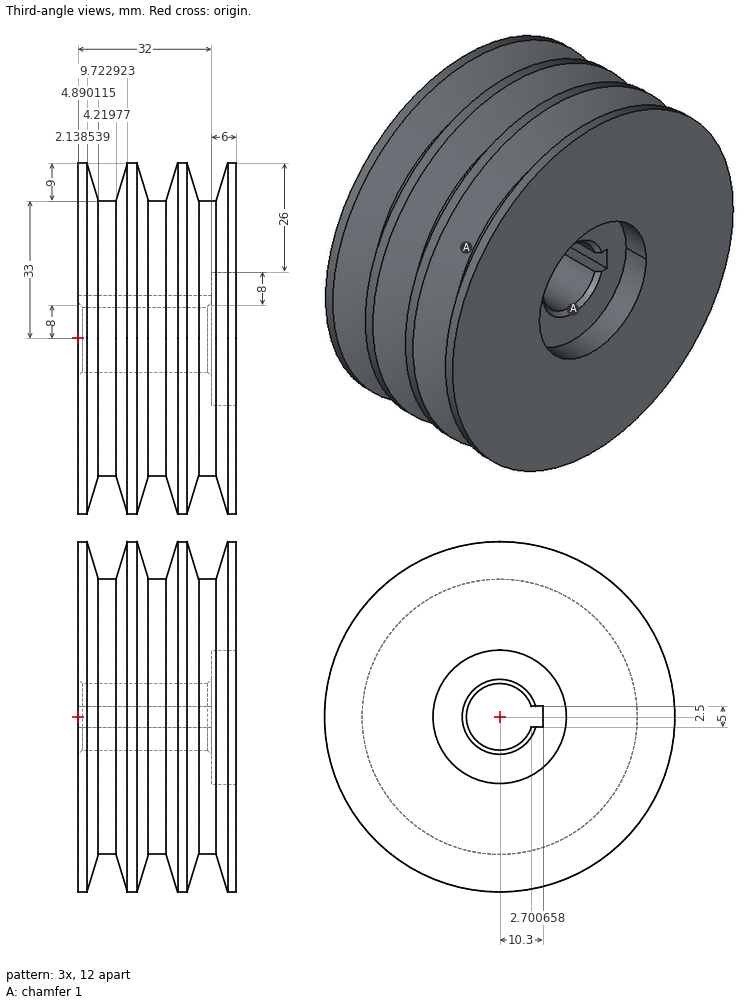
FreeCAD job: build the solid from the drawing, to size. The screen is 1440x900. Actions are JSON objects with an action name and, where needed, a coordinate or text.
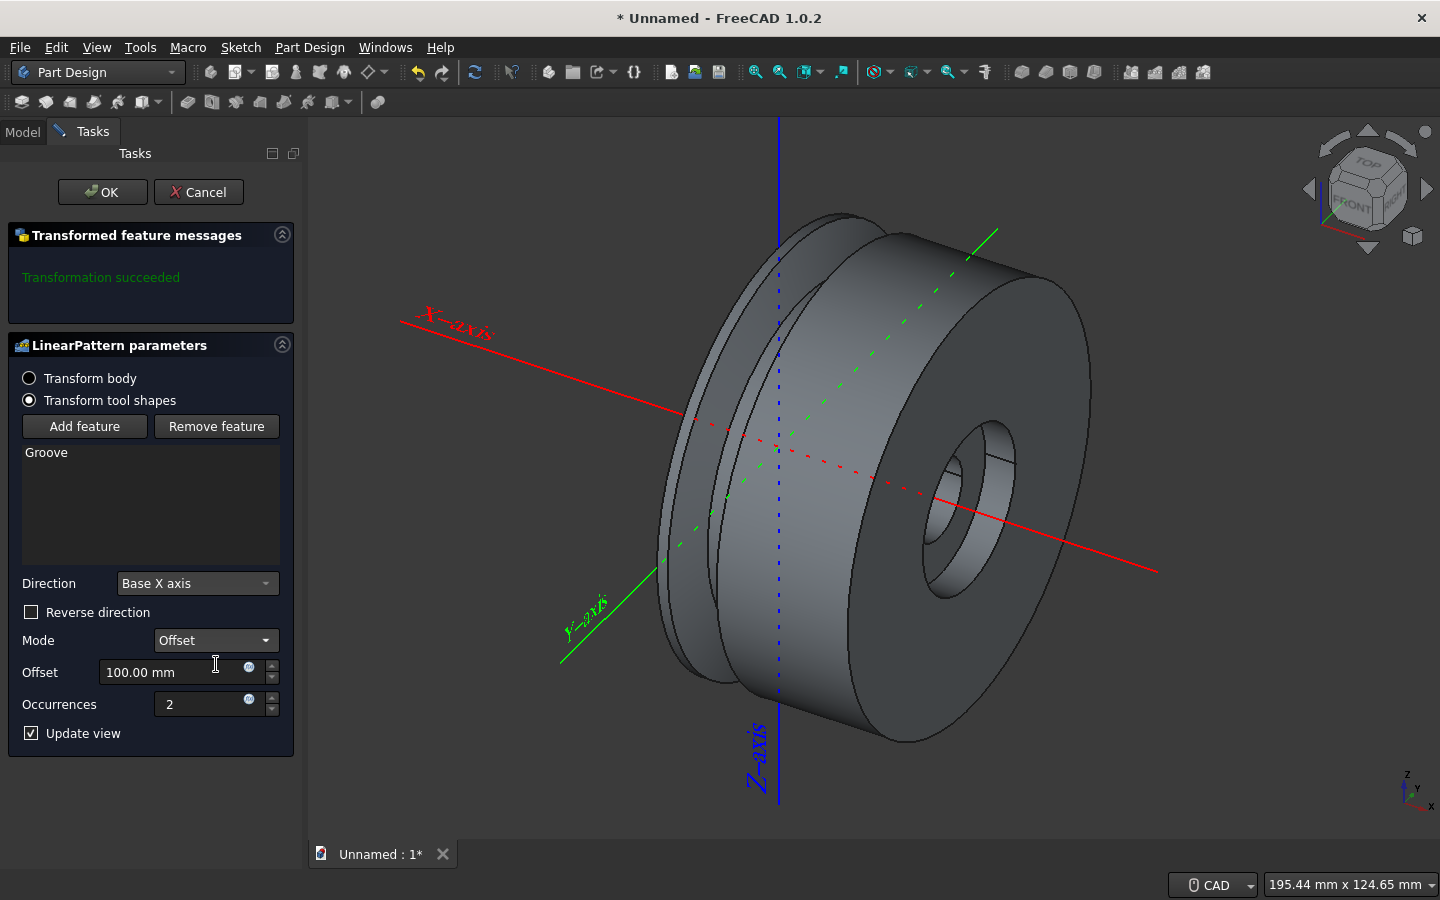
{"action": "triple_click", "coordinate": [182, 672]}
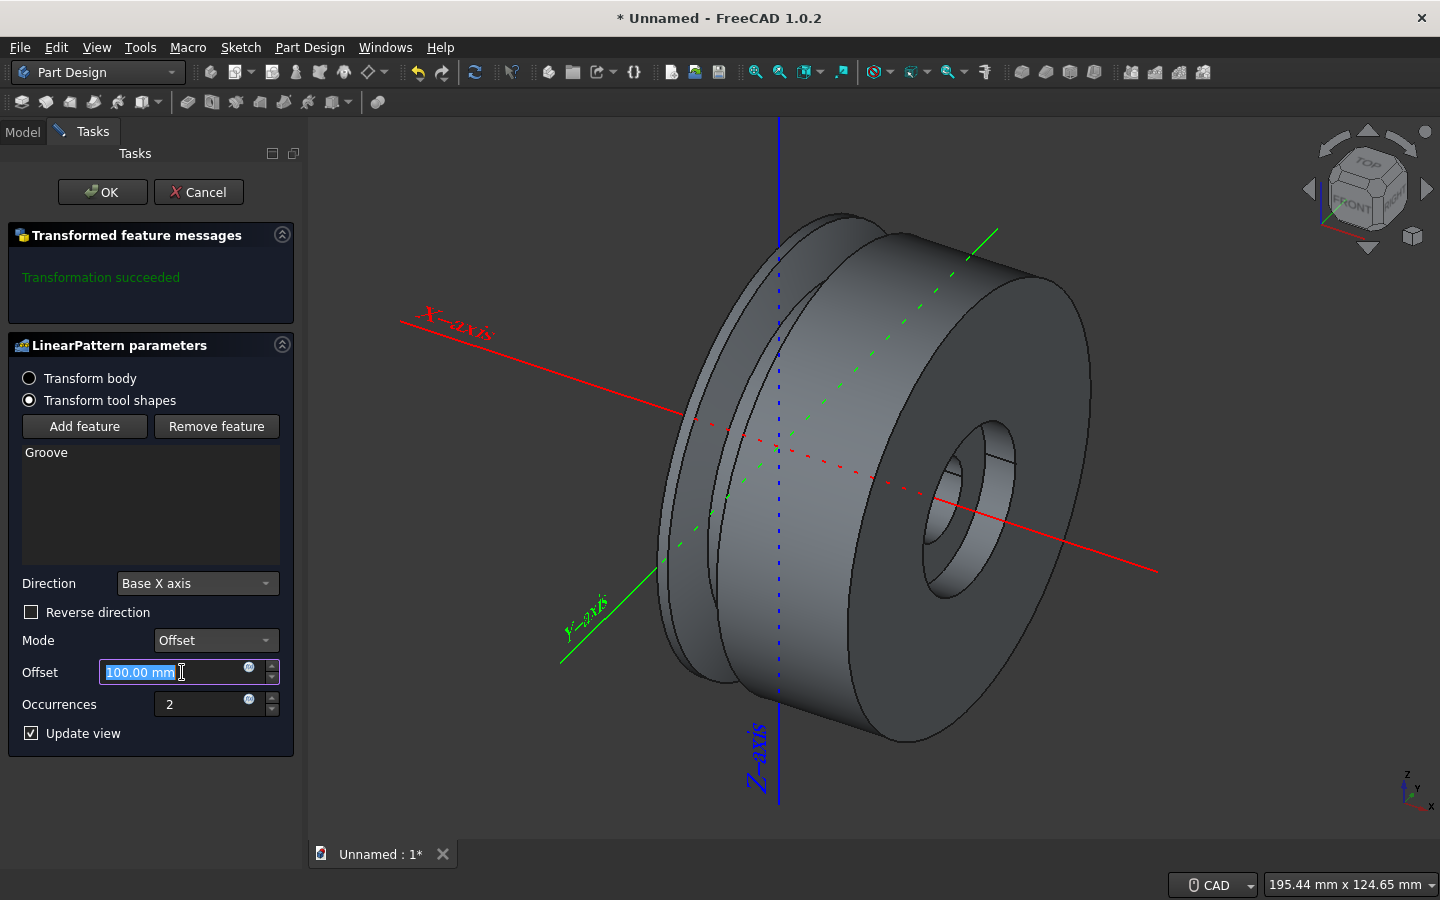
{"action": "type", "text": "12"}
{"action": "key", "text": "Tab"}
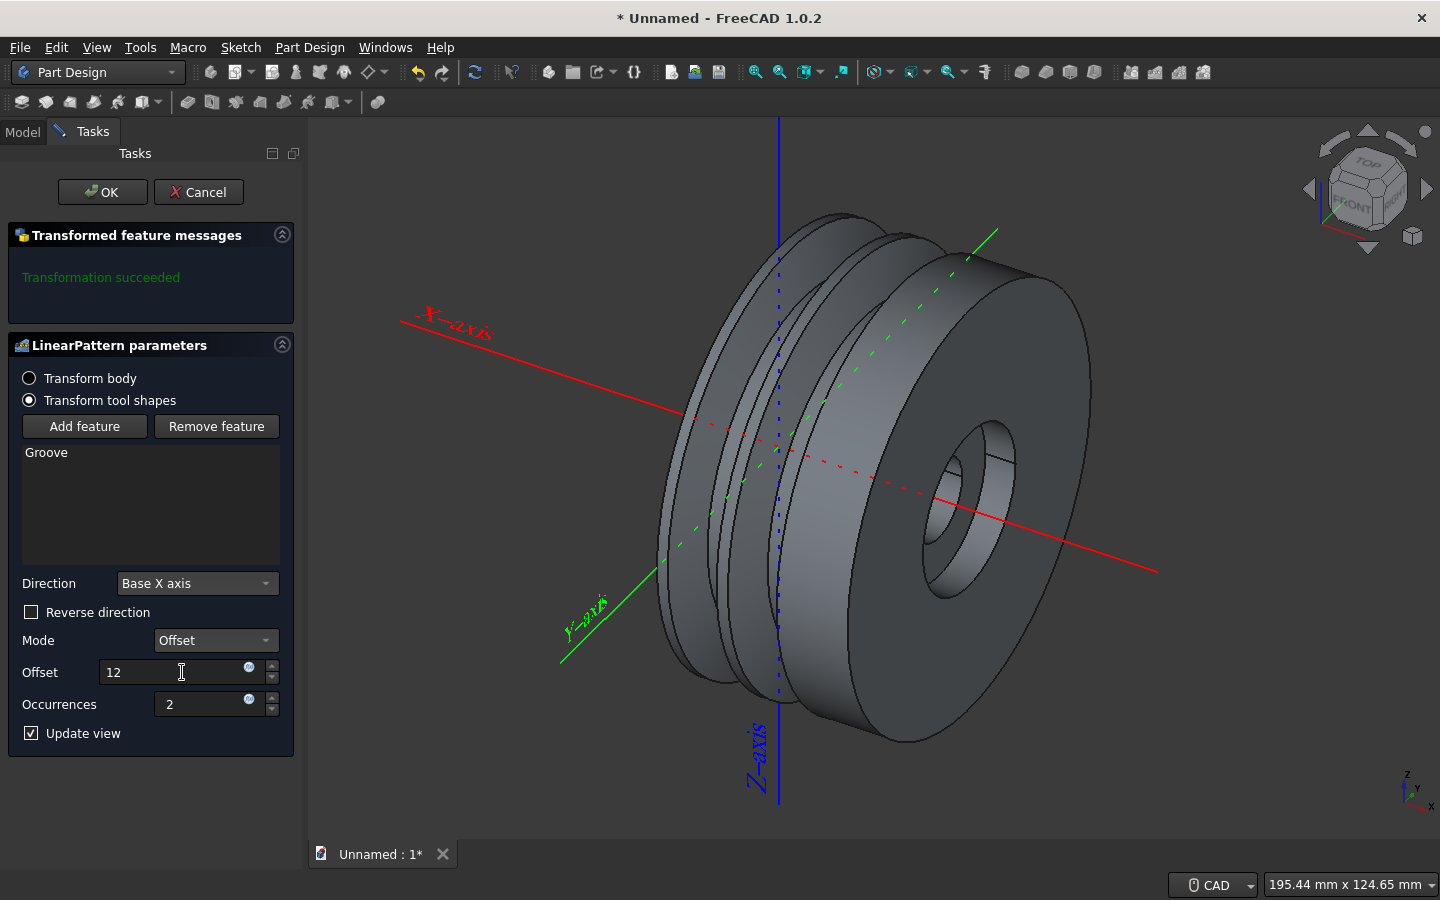
{"action": "triple_click", "coordinate": [209, 704]}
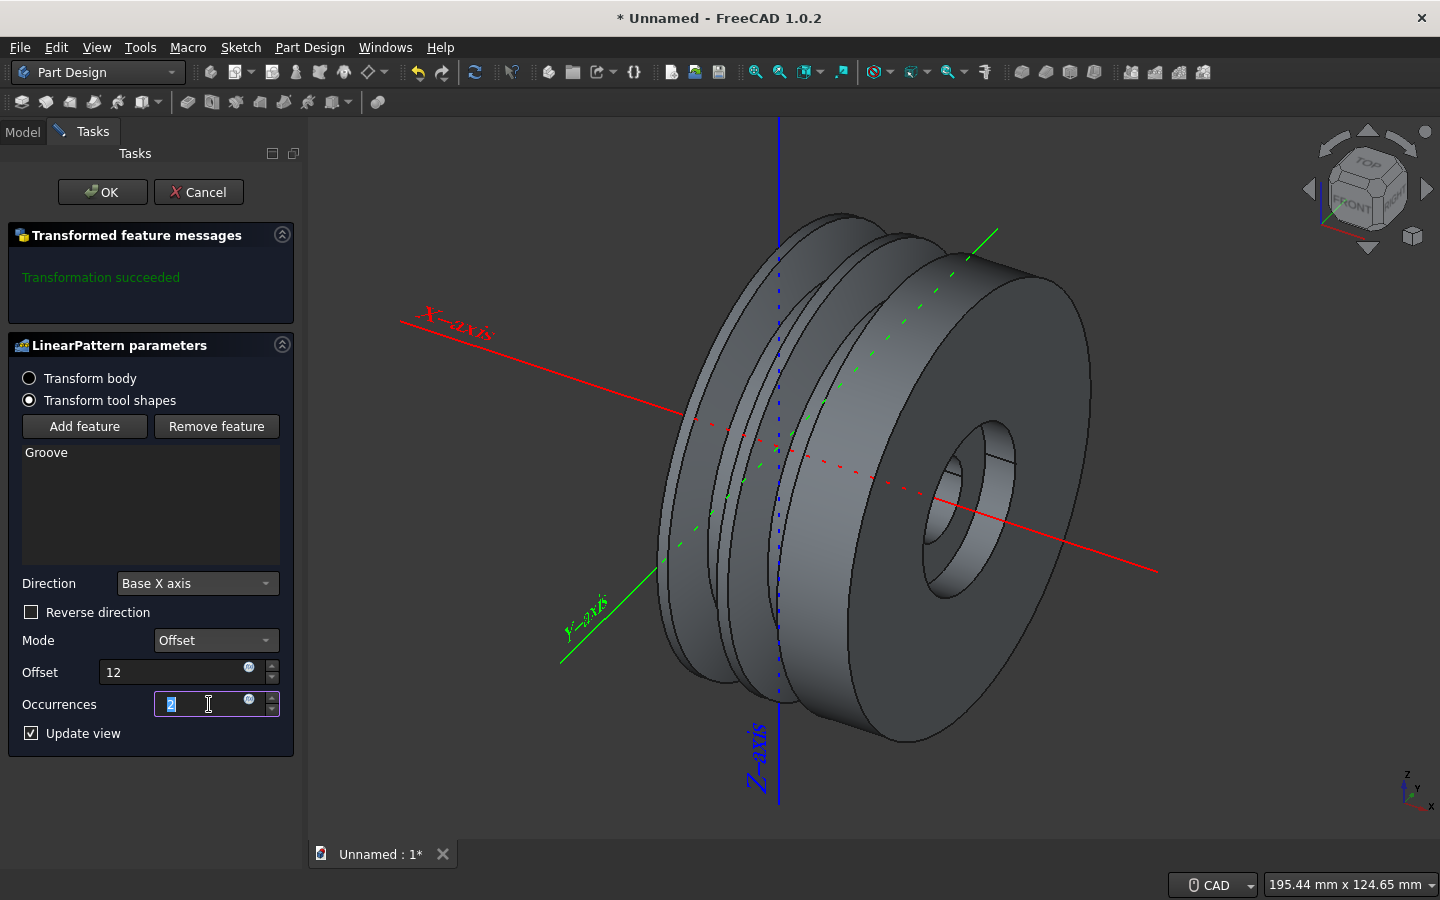
{"action": "type", "text": "3"}
{"action": "key", "text": "Tab"}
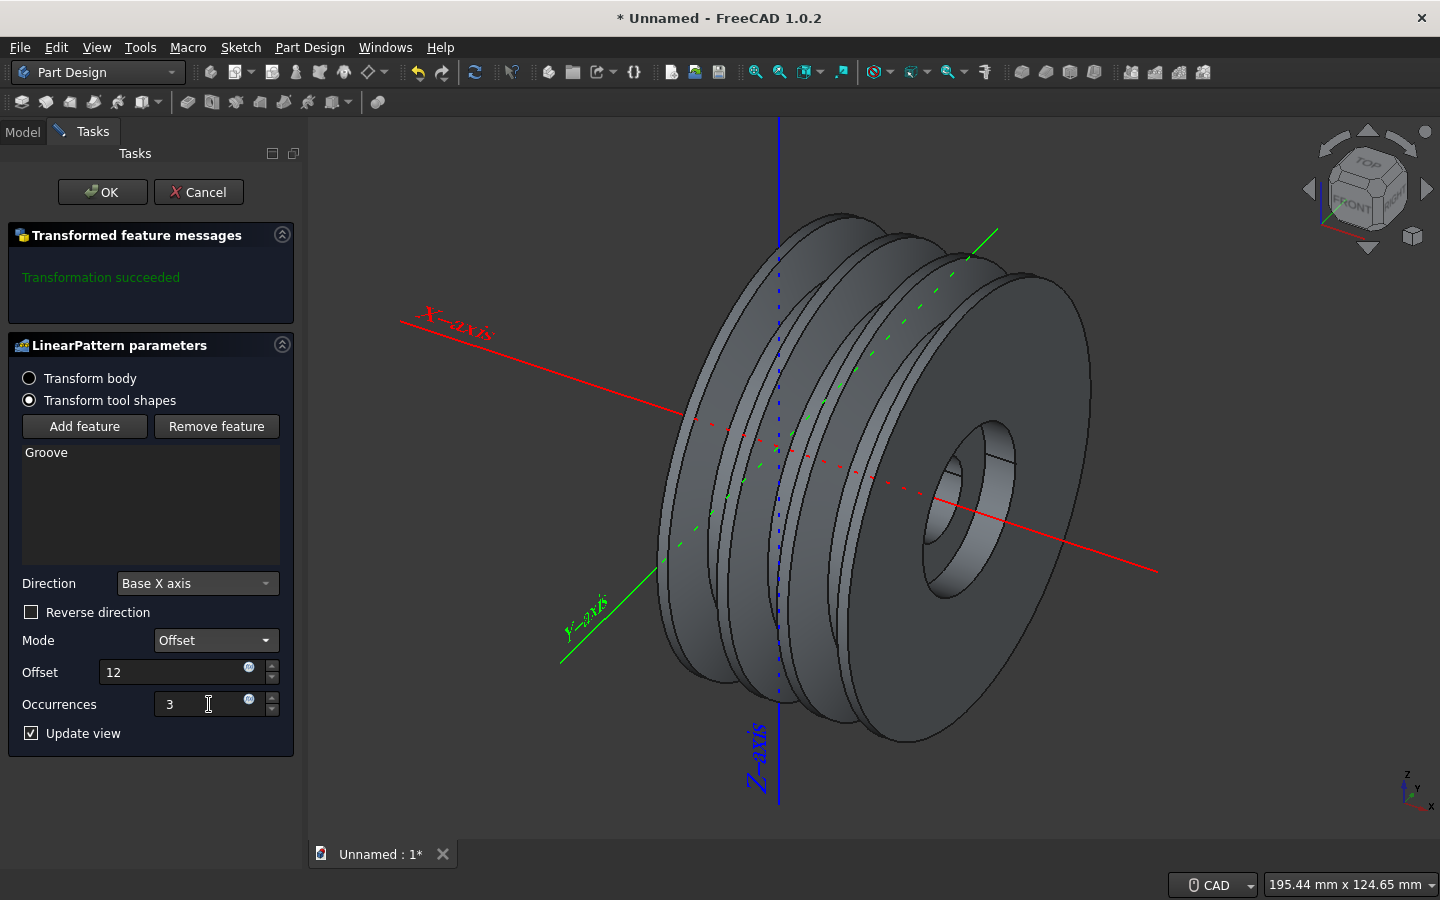
{"action": "left_click", "coordinate": [103, 192]}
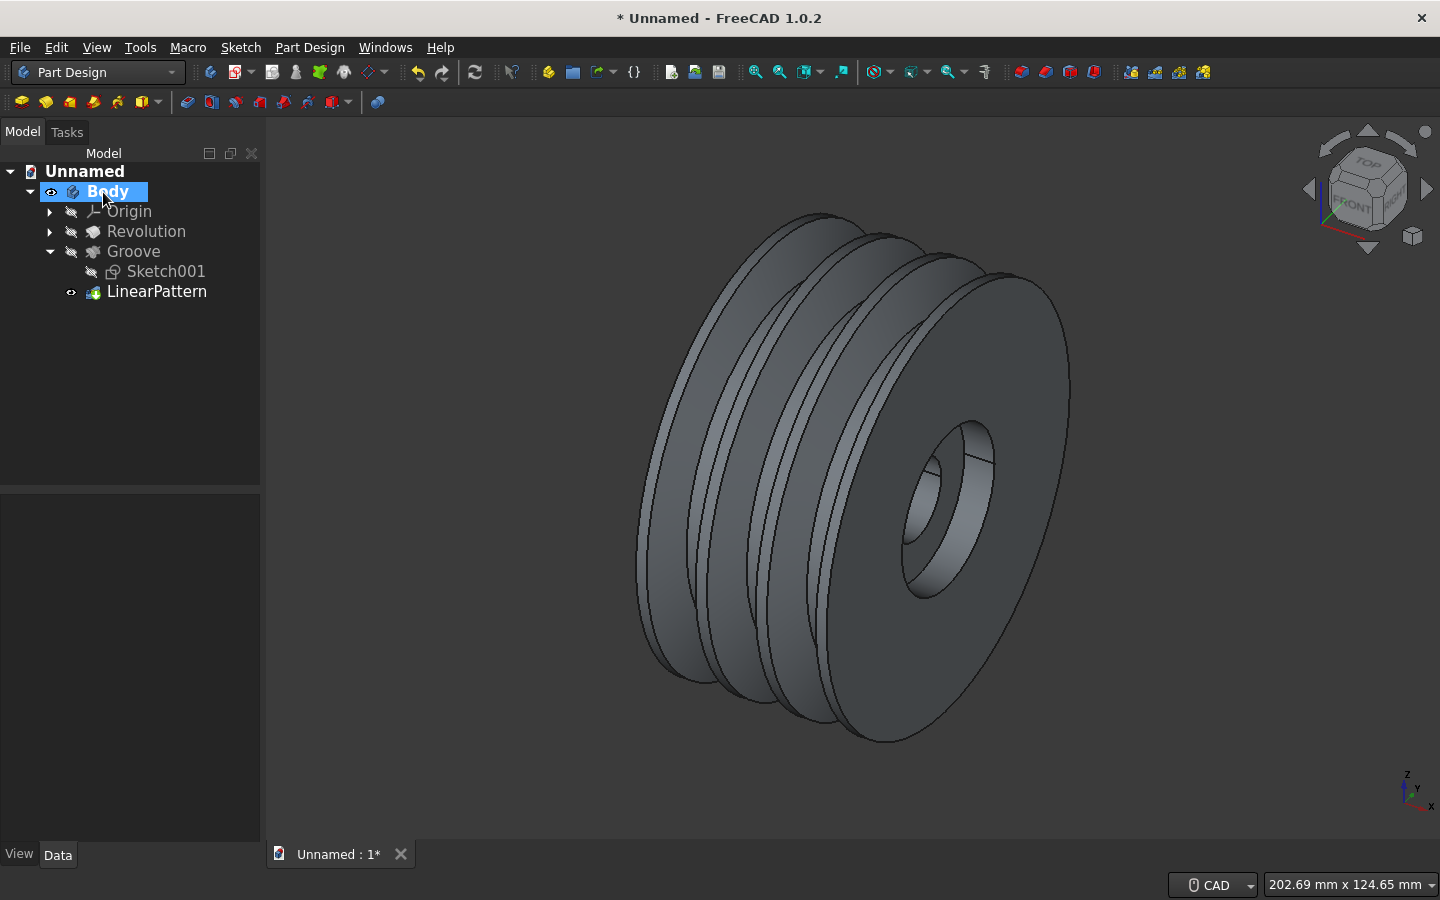
{"action": "left_click", "coordinate": [911, 542]}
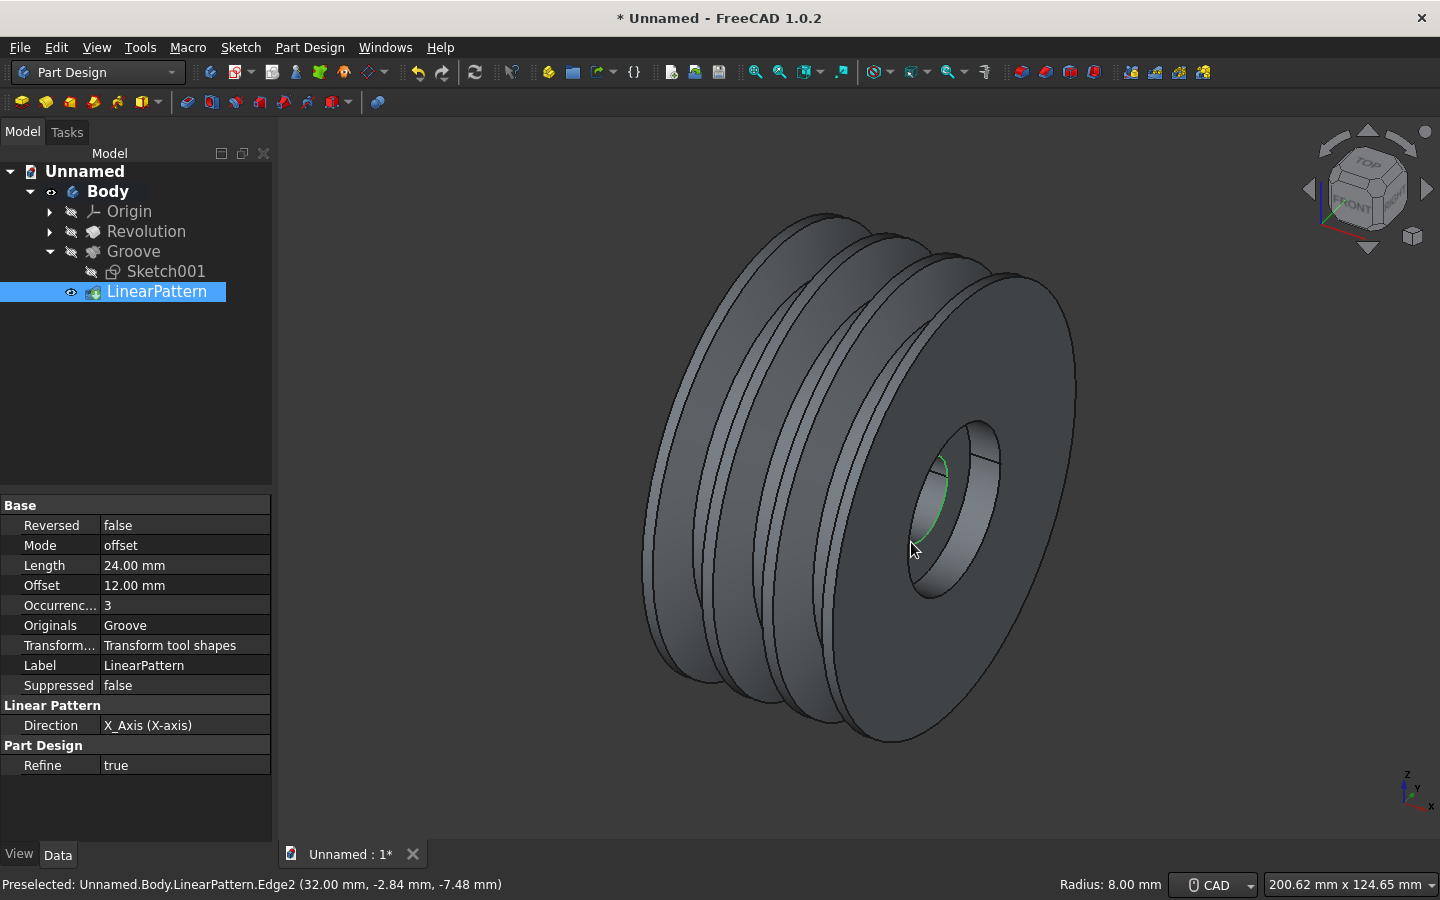
{"action": "key", "text": "0"}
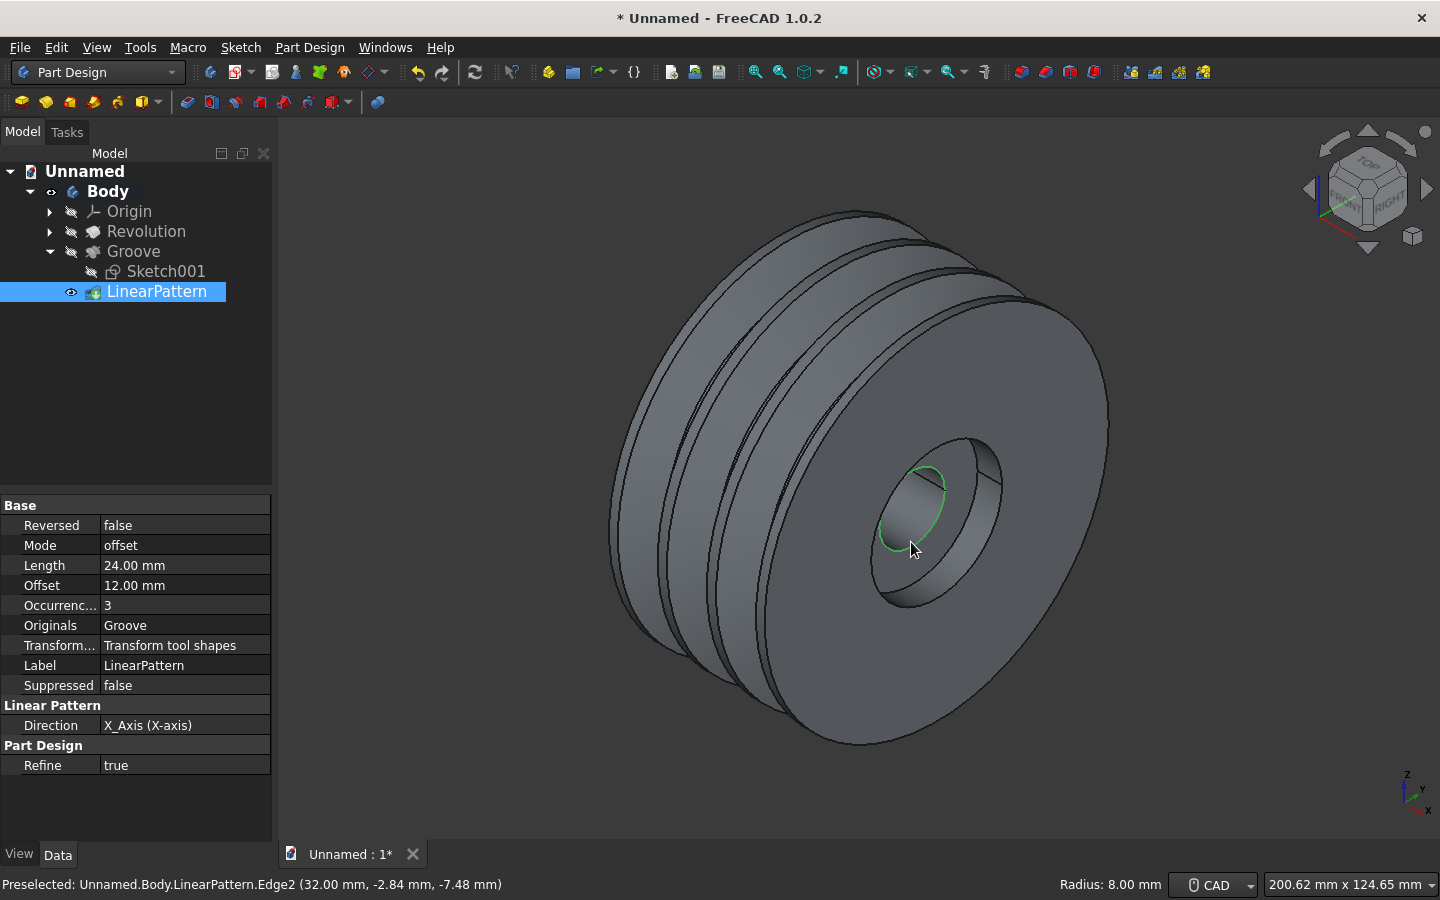
{"action": "key", "text": "2"}